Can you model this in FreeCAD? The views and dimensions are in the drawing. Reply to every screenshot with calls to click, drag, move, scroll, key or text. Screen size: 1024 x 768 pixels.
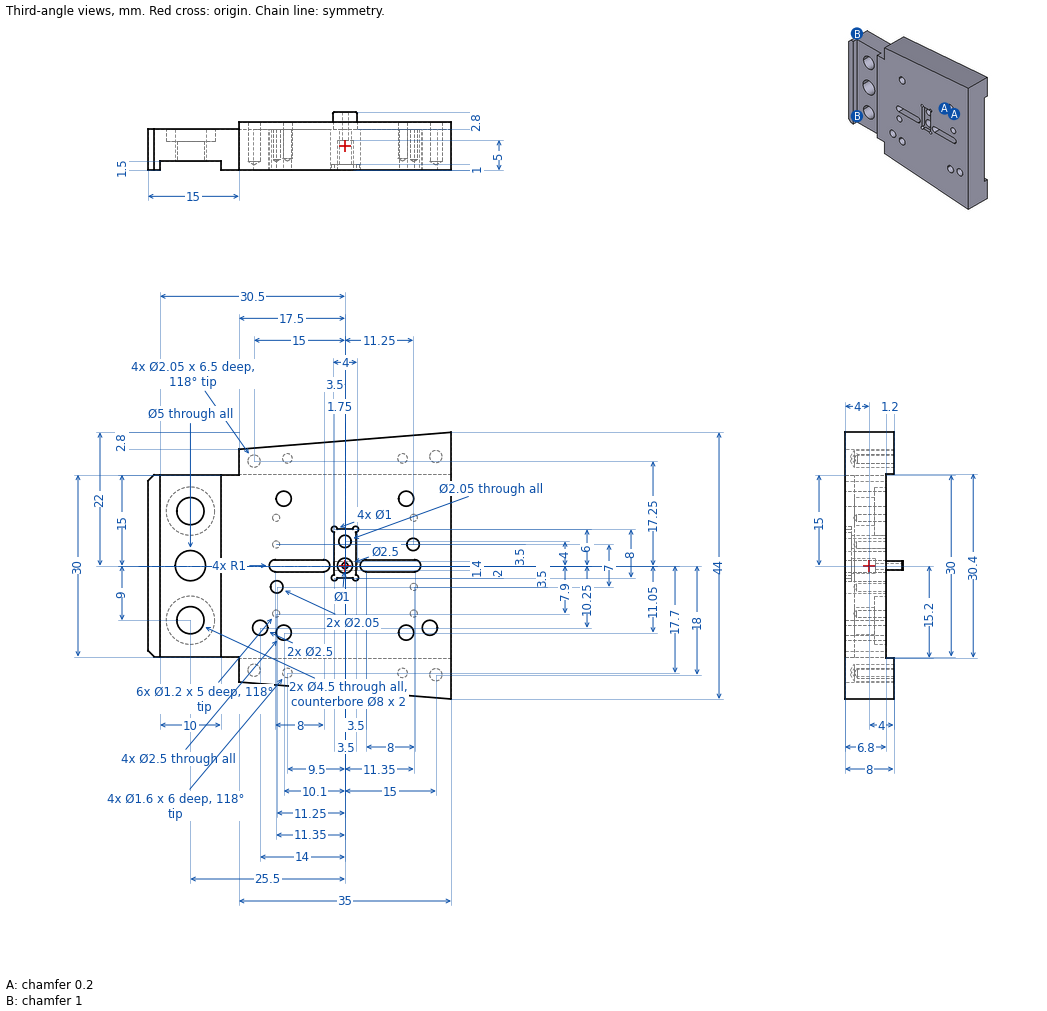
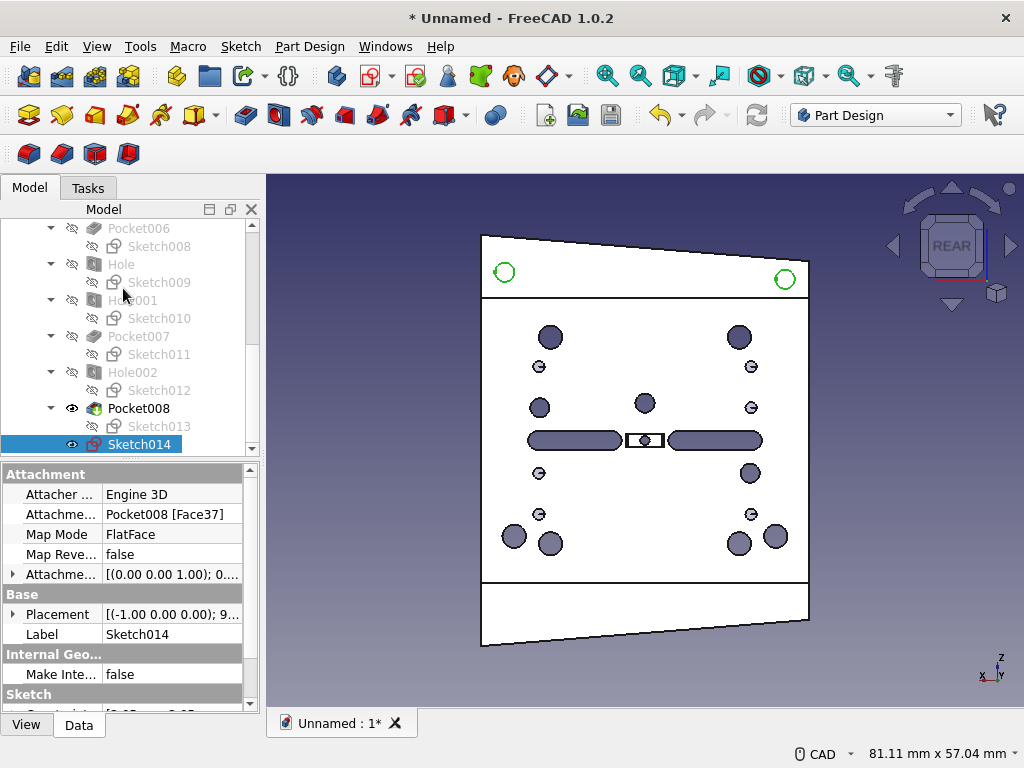
click(279, 116)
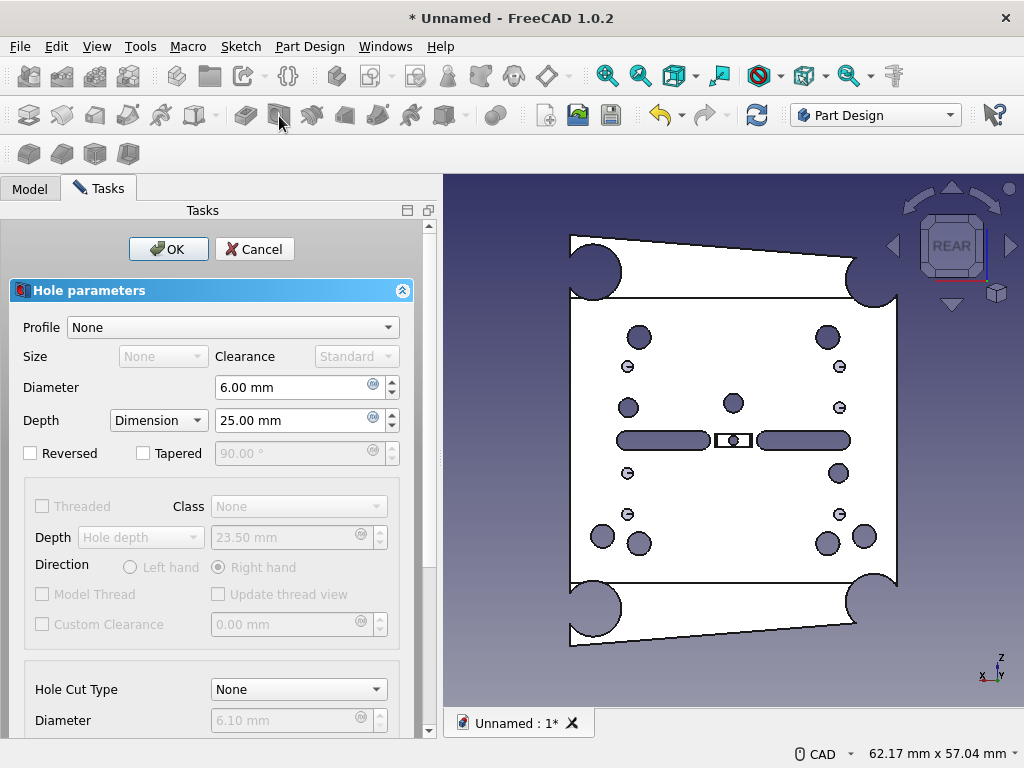
triple_click(300, 388)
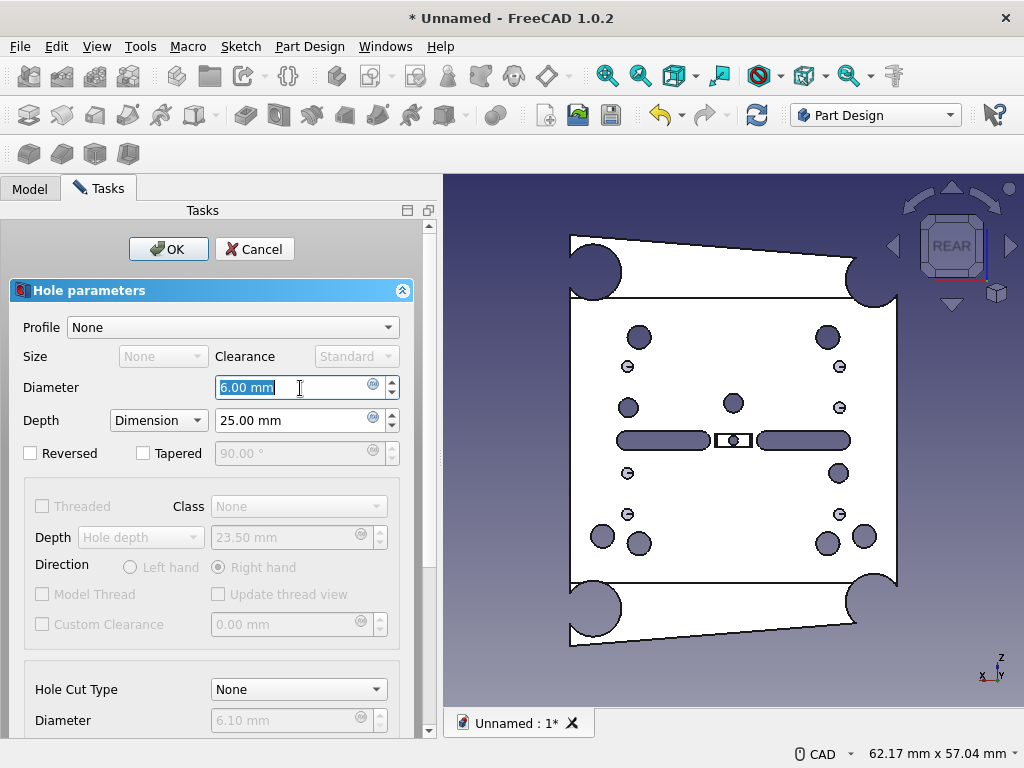
text(2.05)
key(Tab)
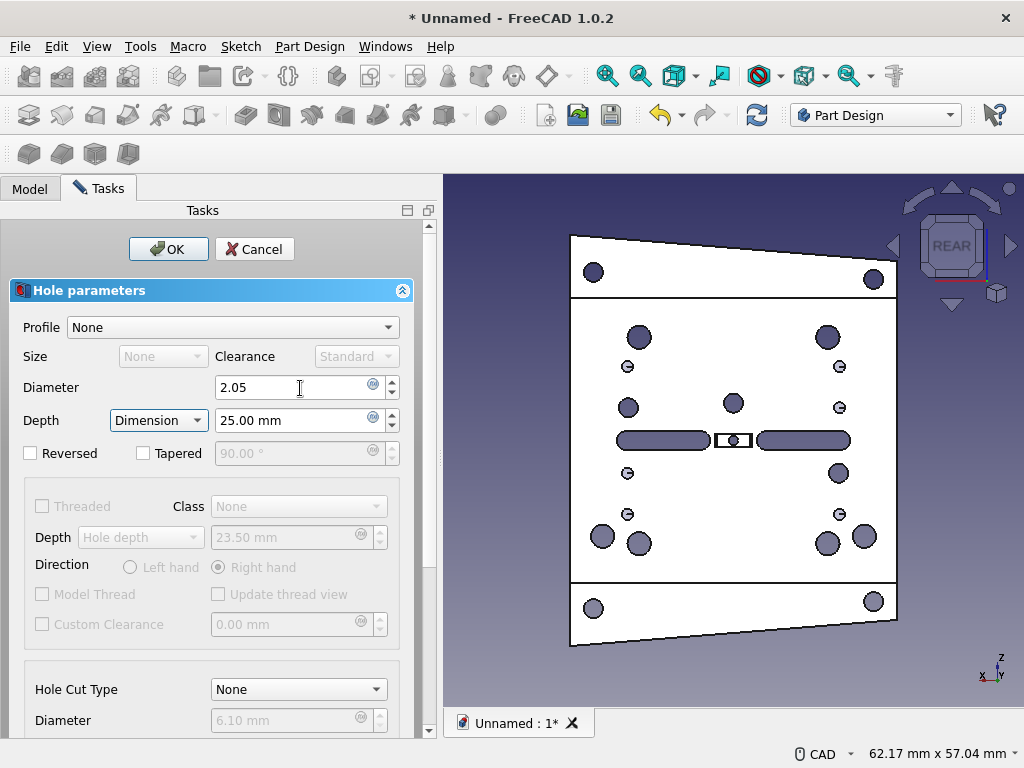
triple_click(300, 420)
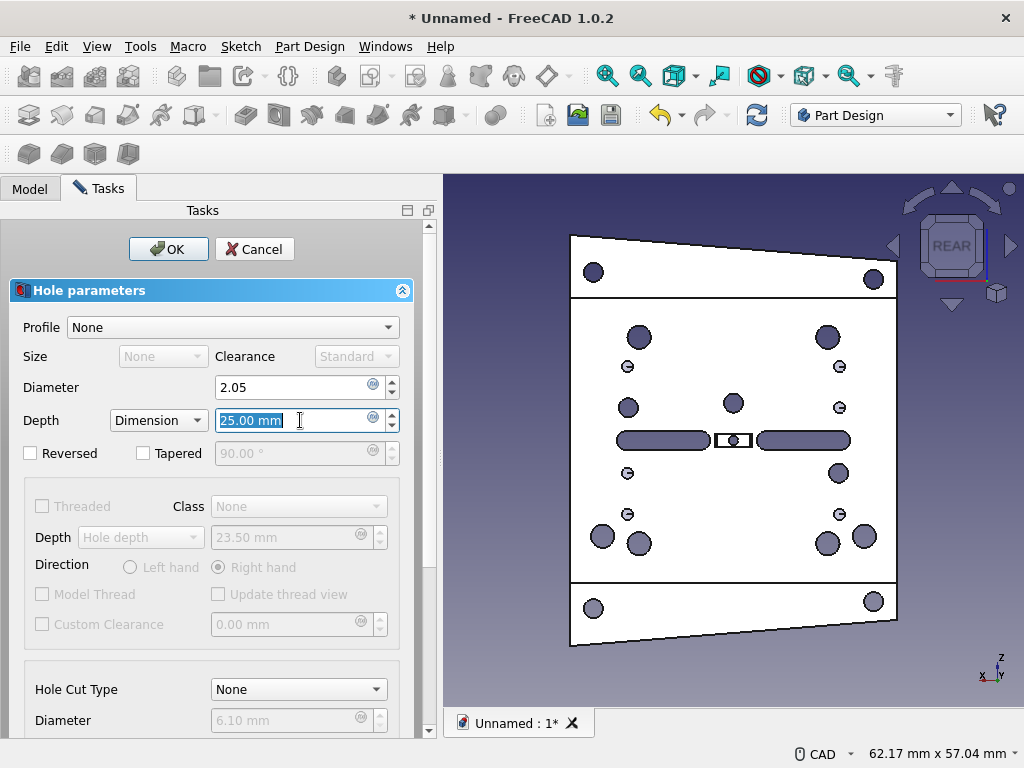
text(6.5)
key(Tab)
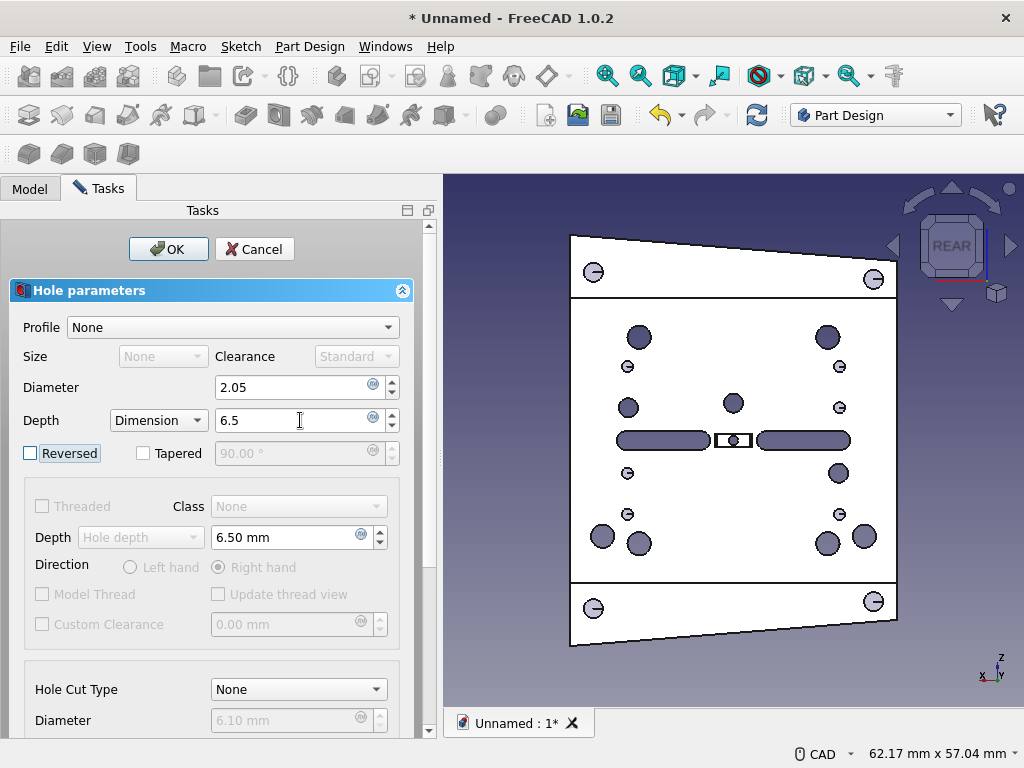
click(169, 249)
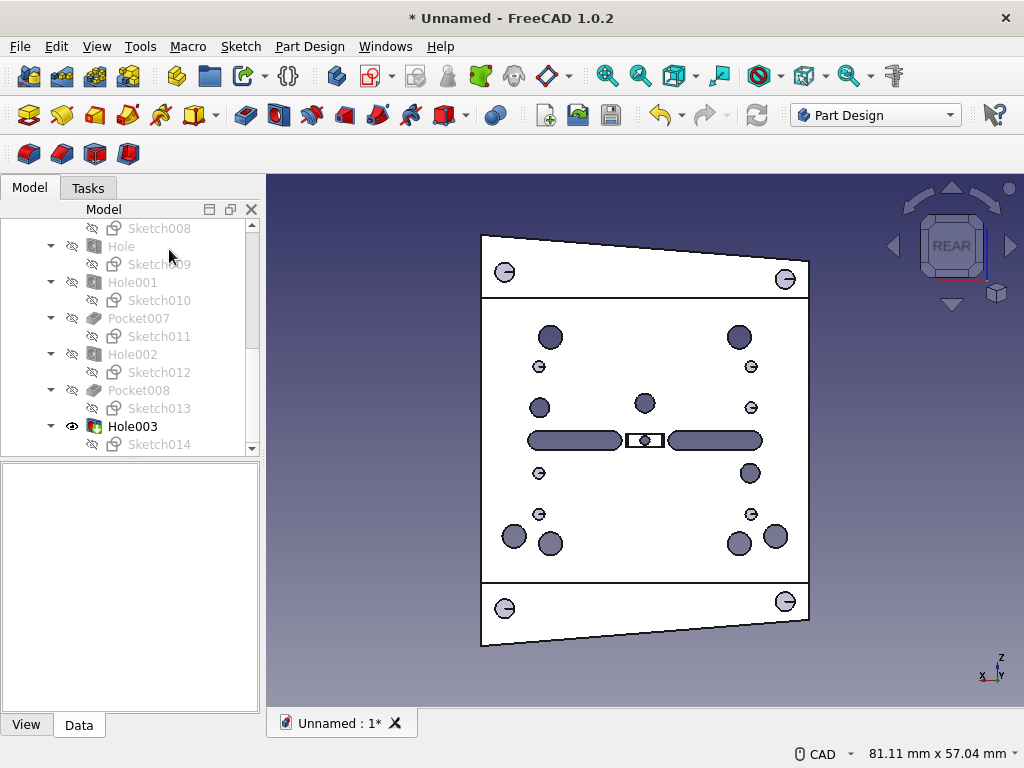
click(552, 613)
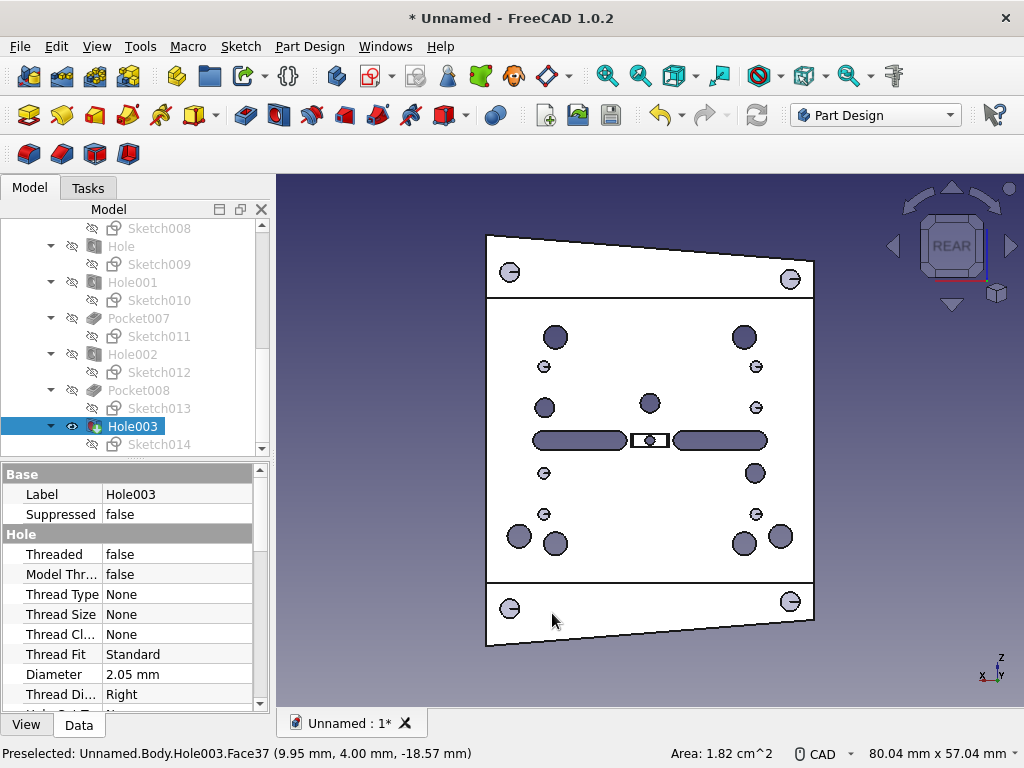
click(370, 76)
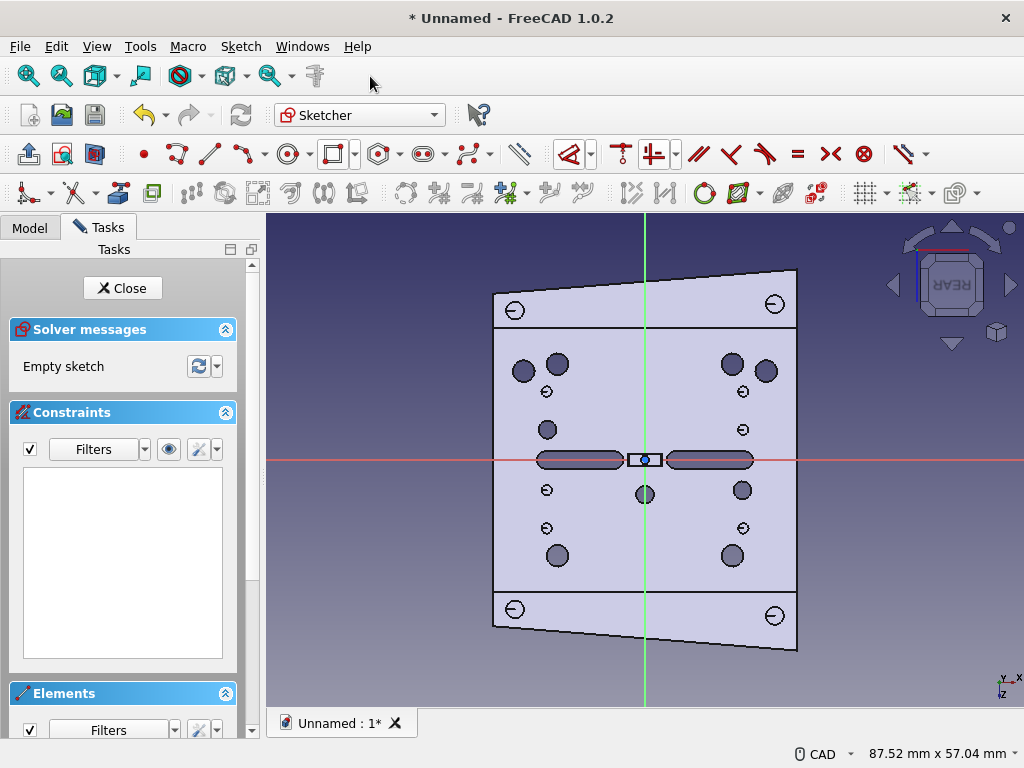
click(288, 154)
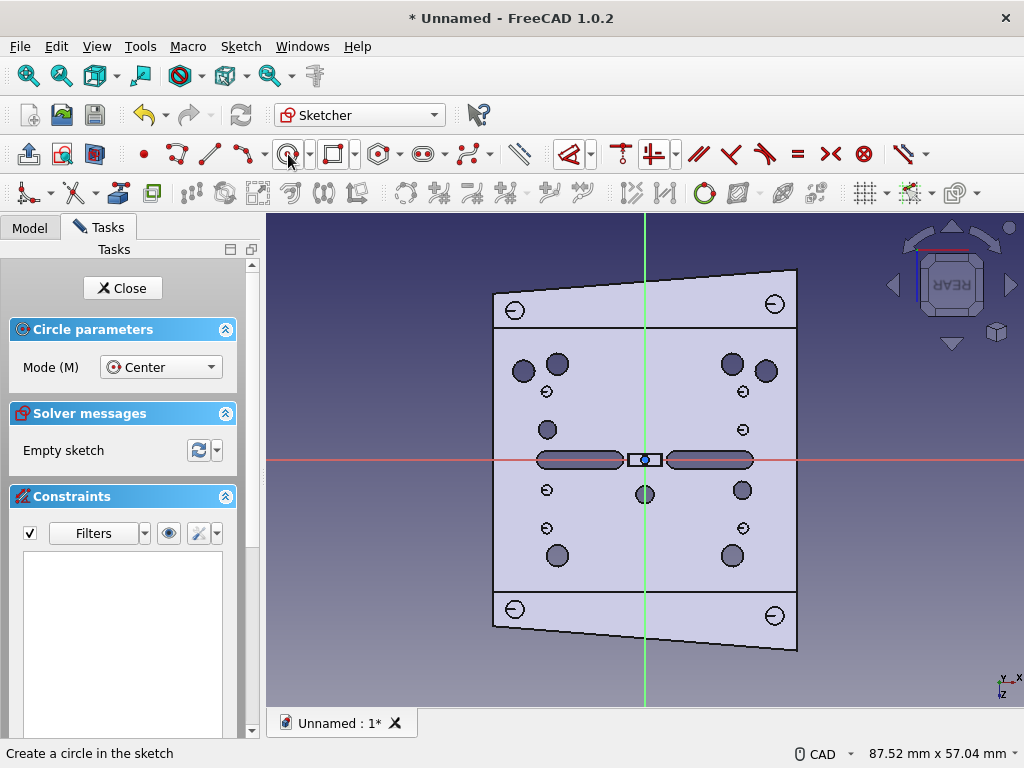
scroll(563, 307, up, 6)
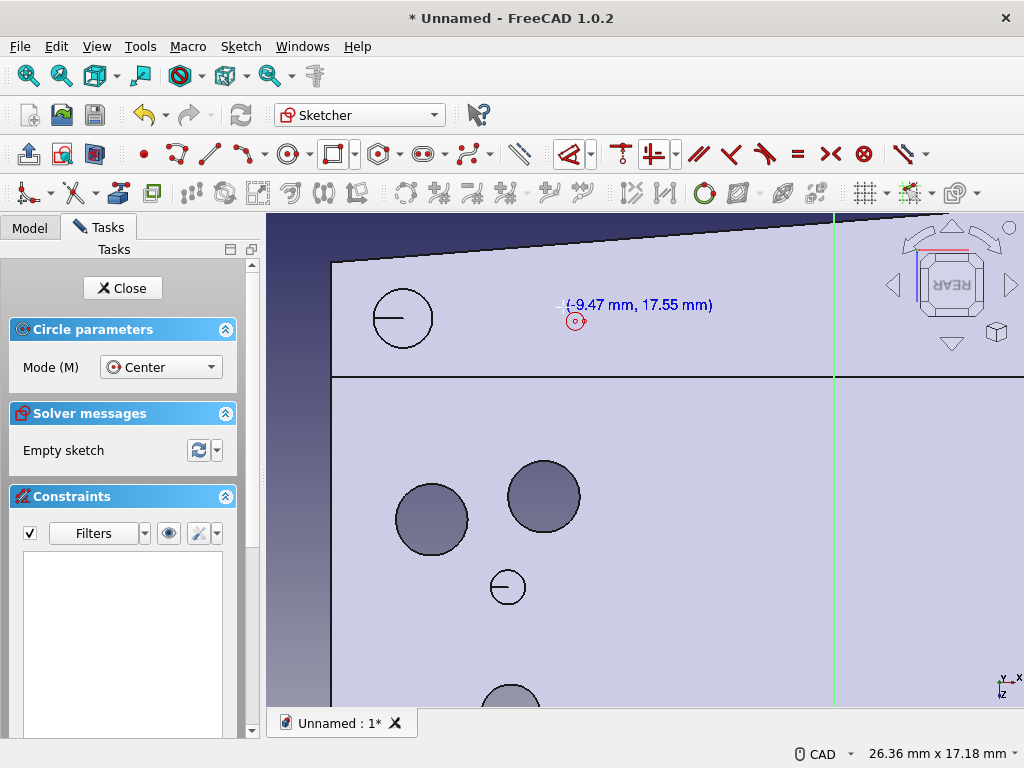
click(561, 306)
move(577, 289)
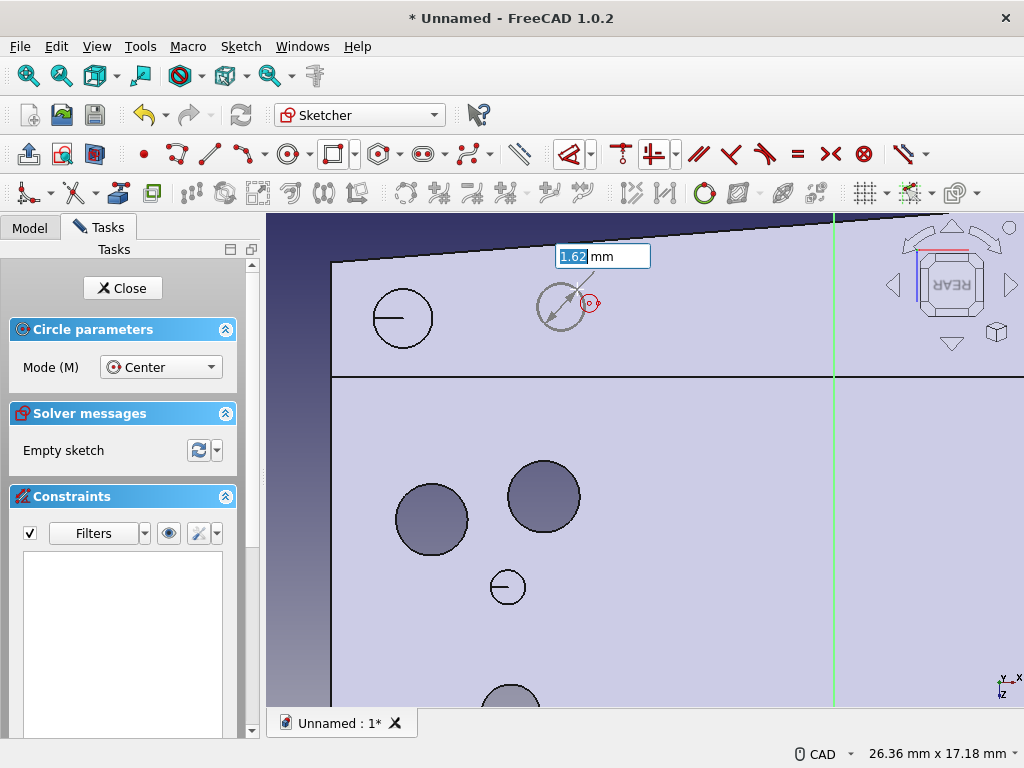
text(1.6)
key(Return)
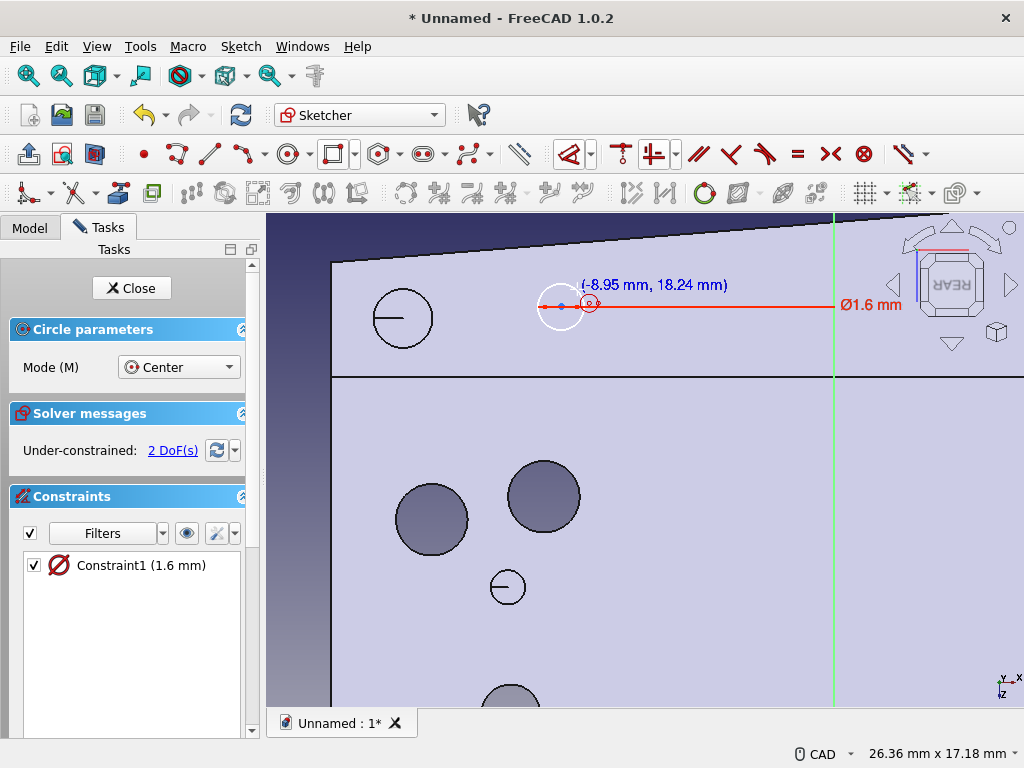
scroll(465, 307, down, 6)